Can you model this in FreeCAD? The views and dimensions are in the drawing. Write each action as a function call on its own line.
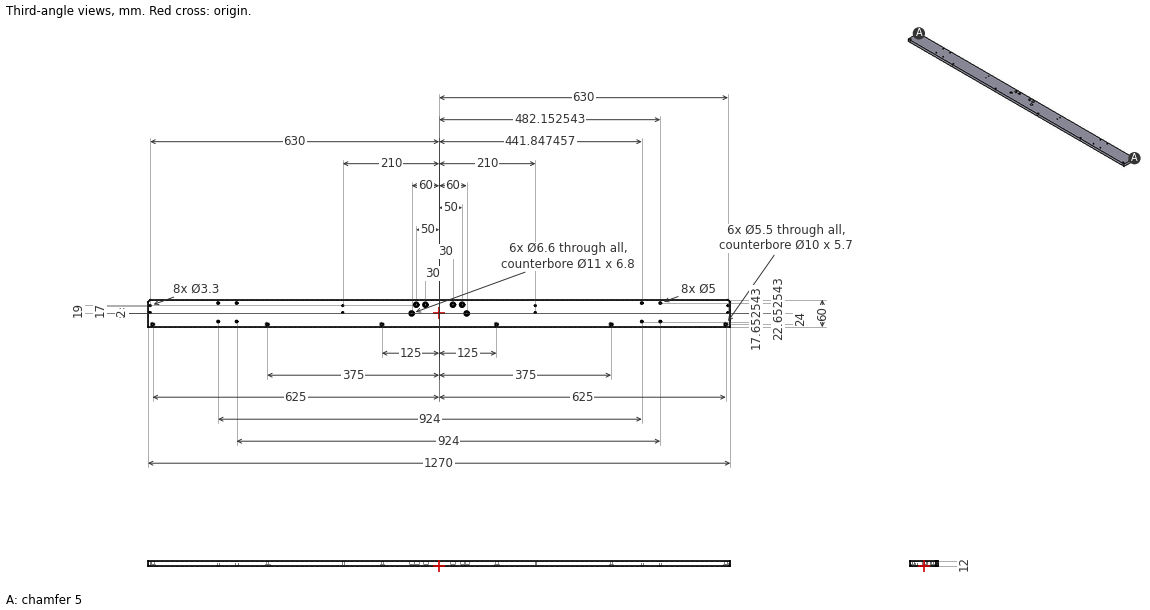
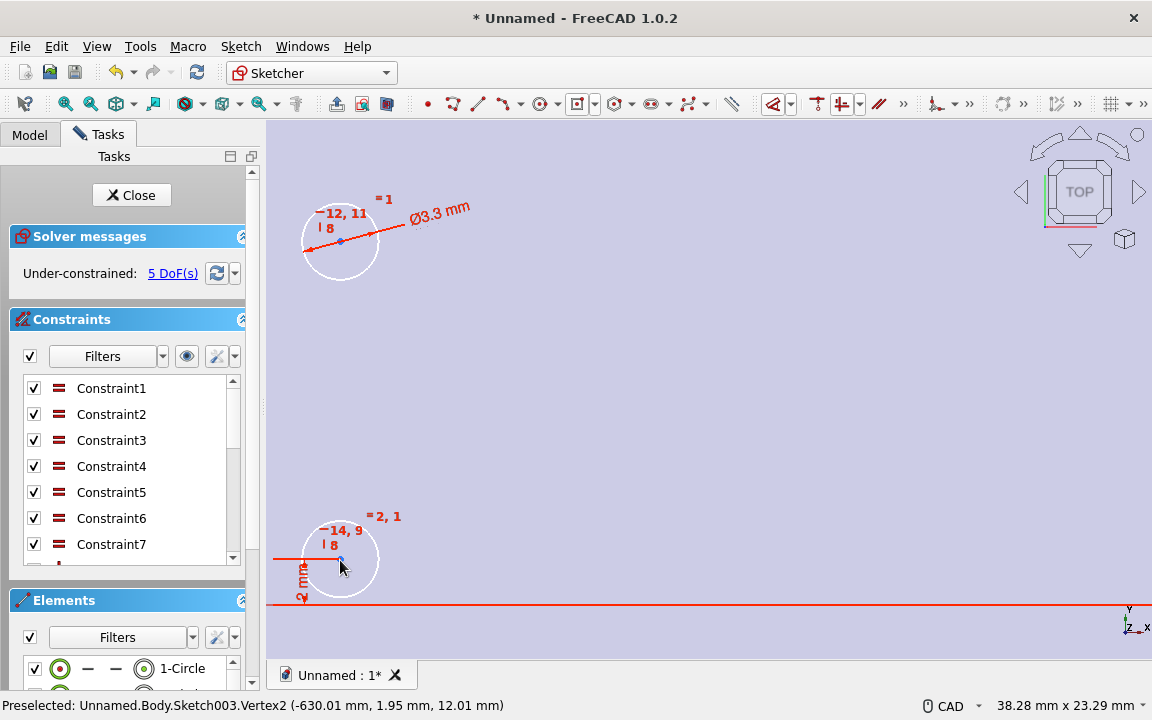
scroll(640, 390, down, 15)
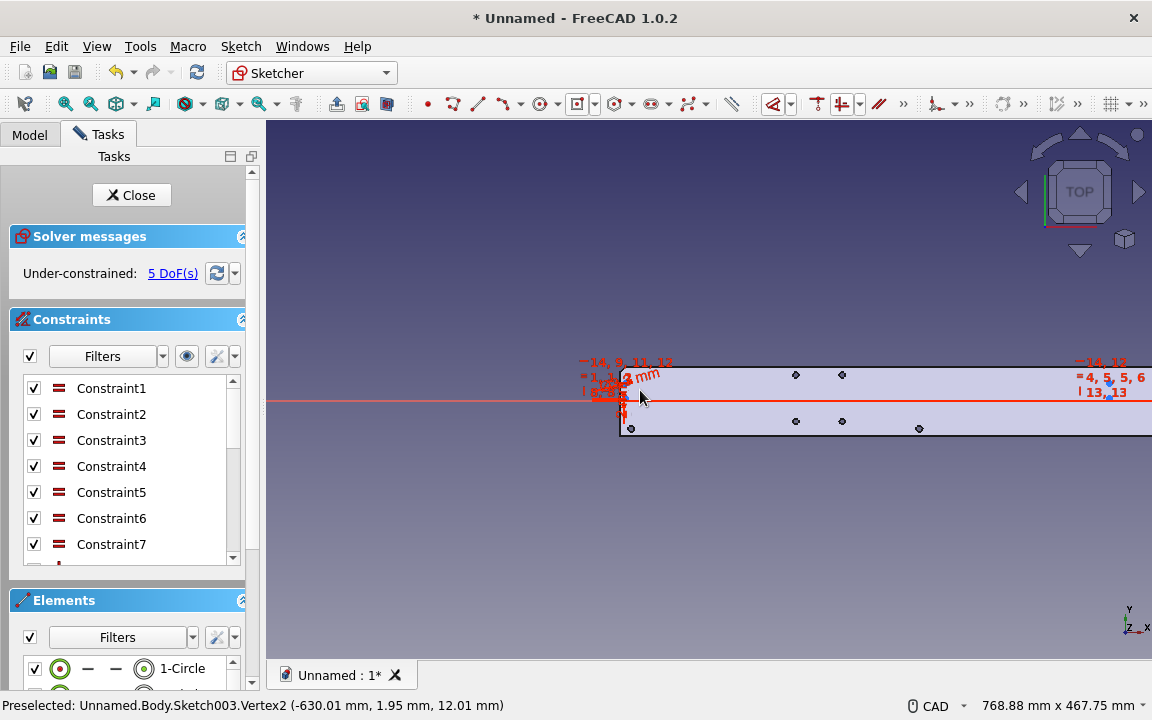
scroll(294, 389, down, 5)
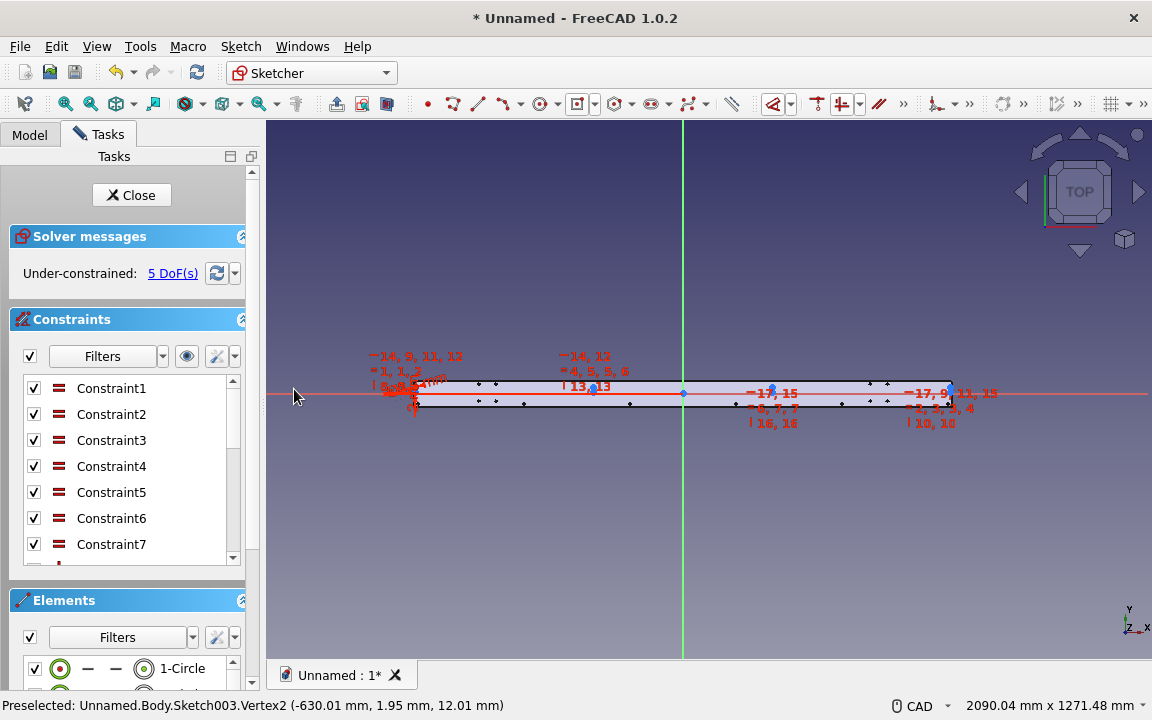
scroll(416, 387, up, 9)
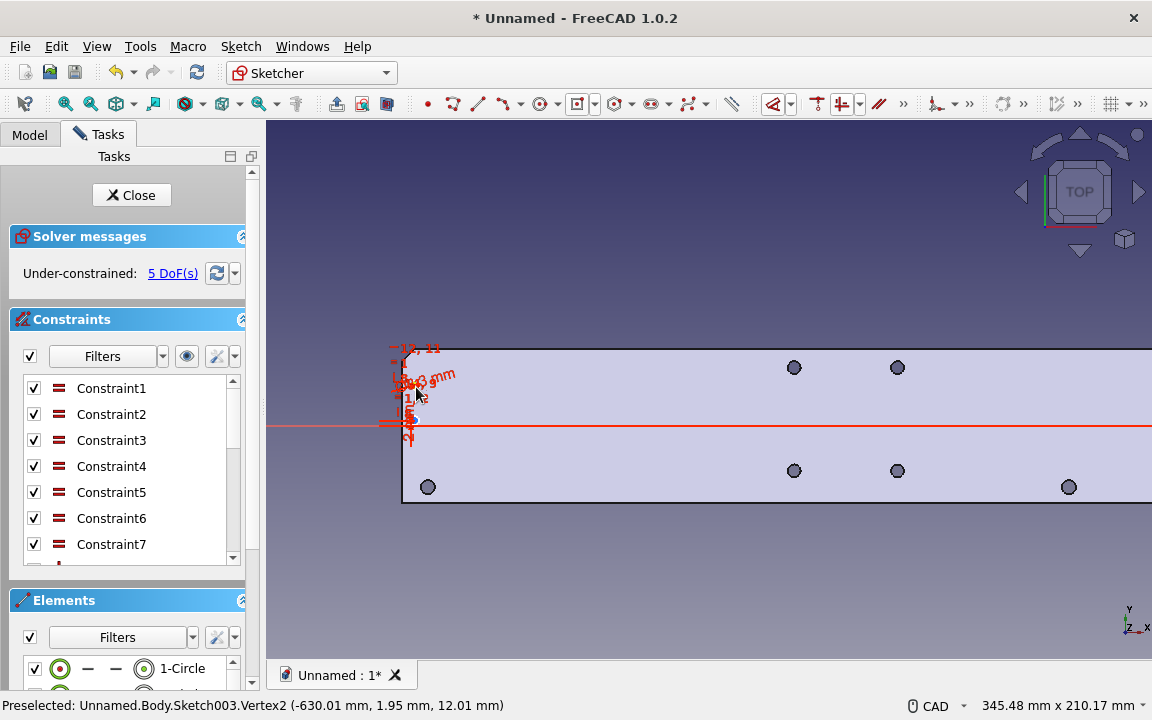
click(415, 385)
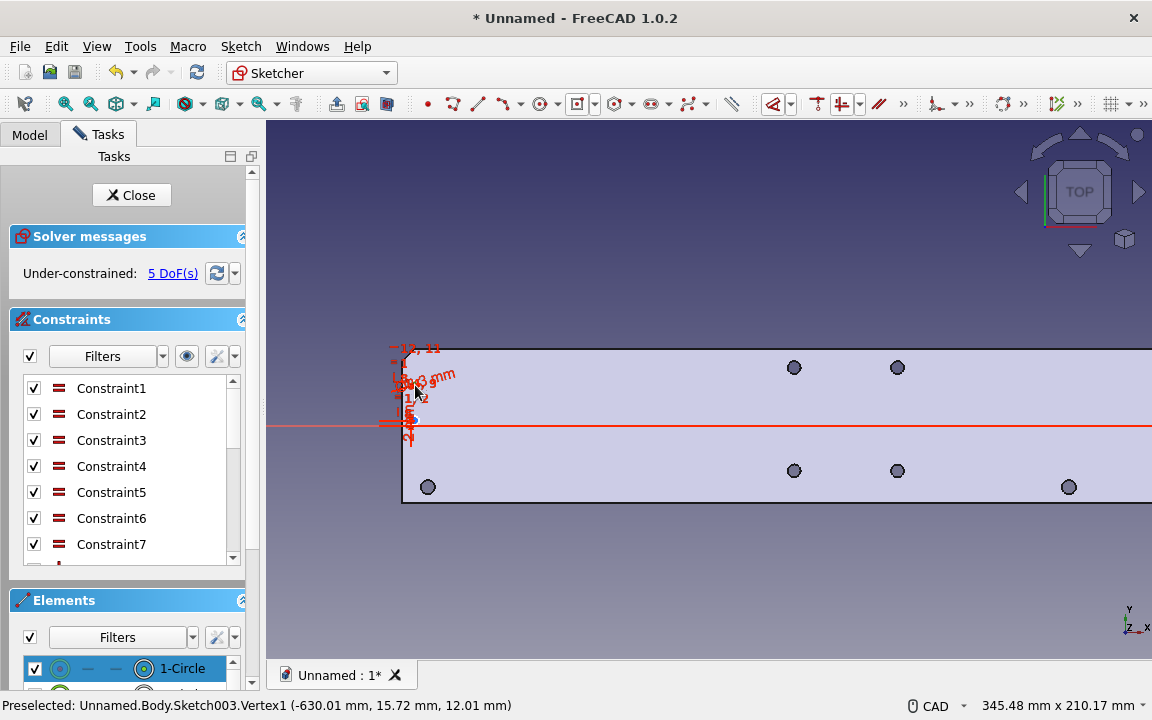
key(i)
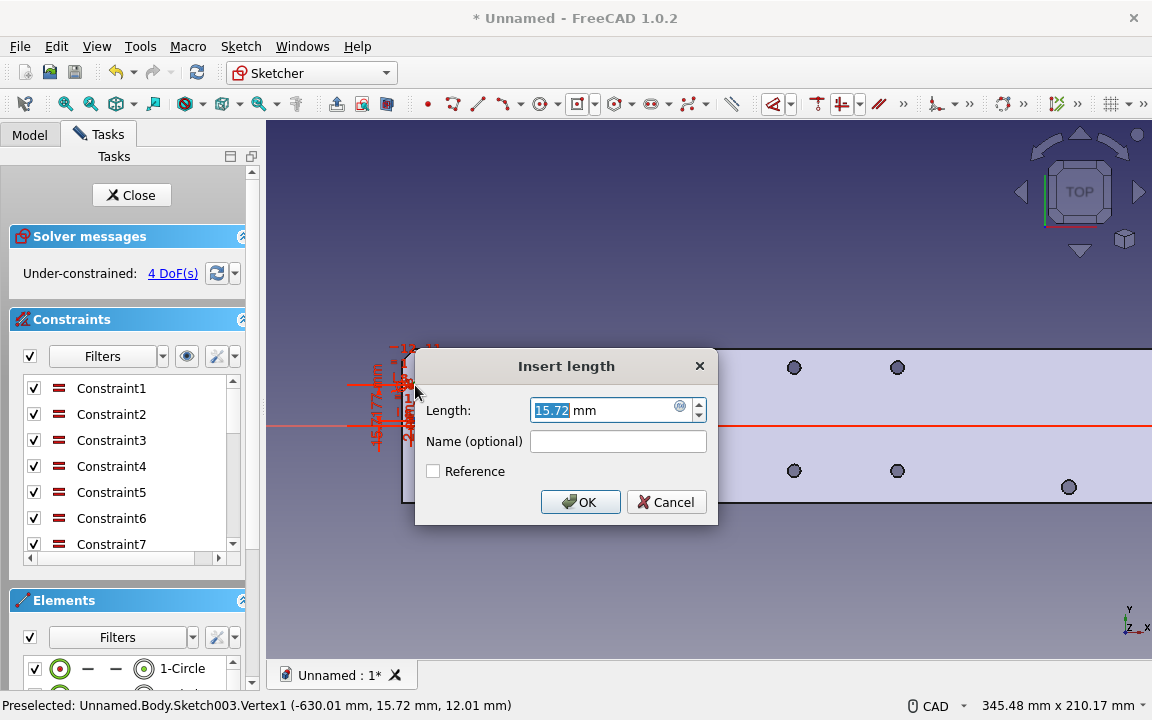
text(17)
key(Return)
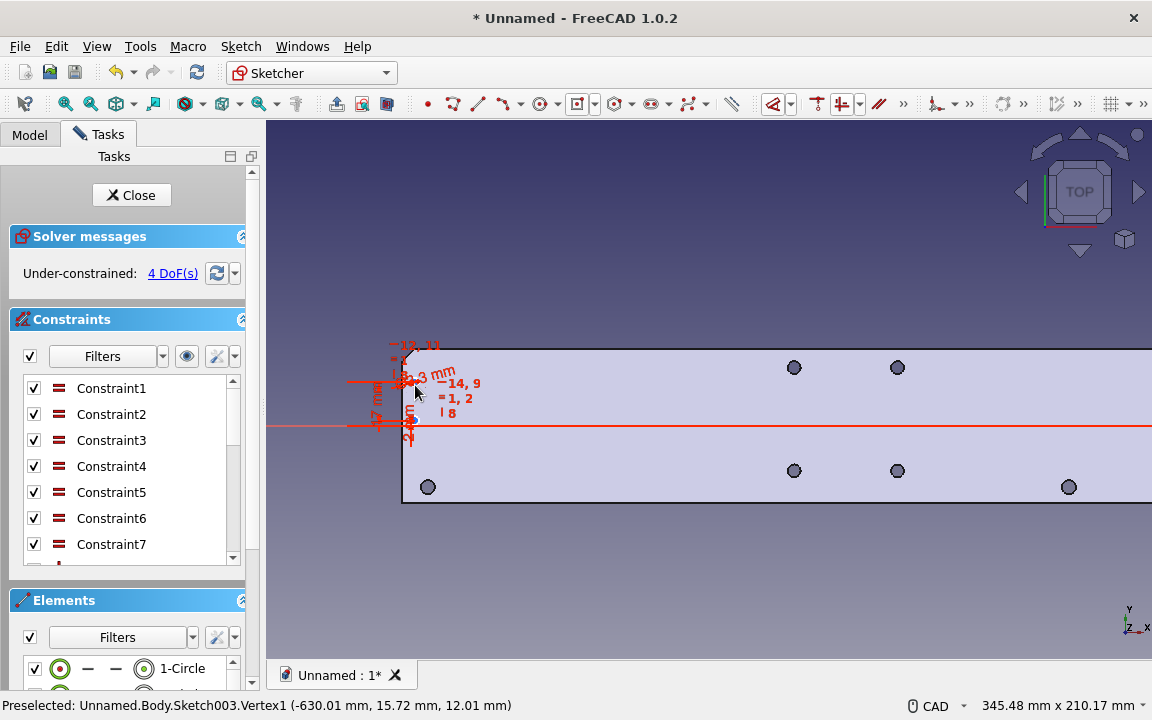
scroll(365, 387, down, 9)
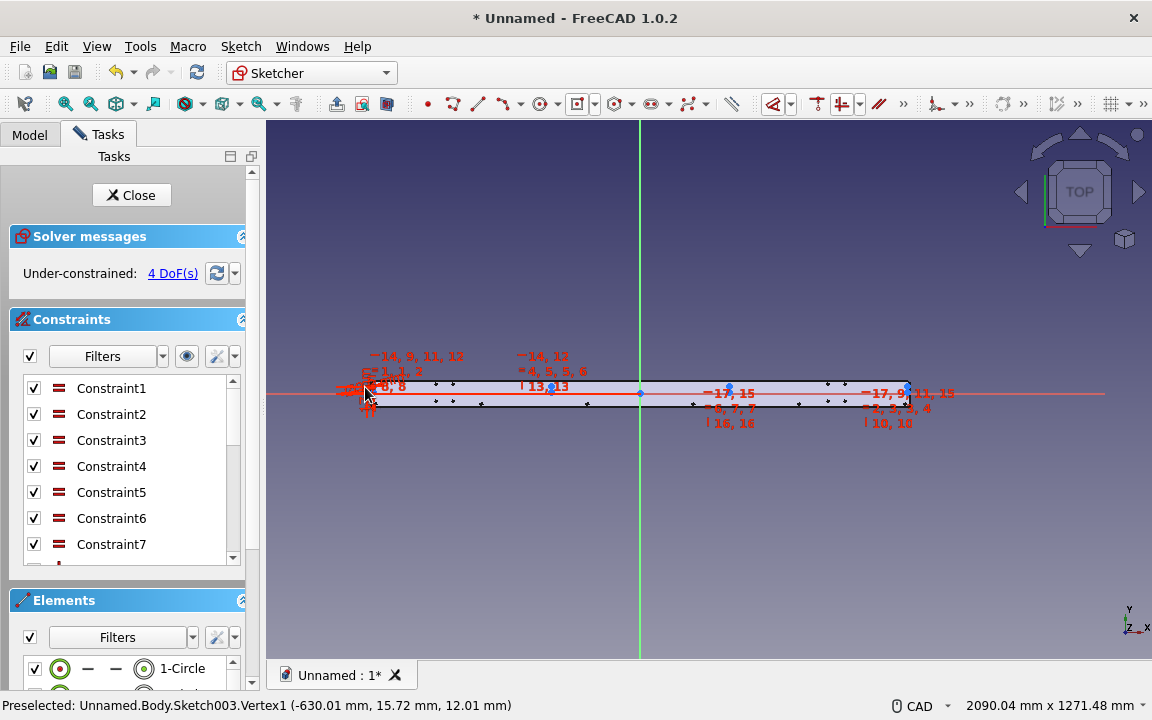
scroll(373, 387, up, 4)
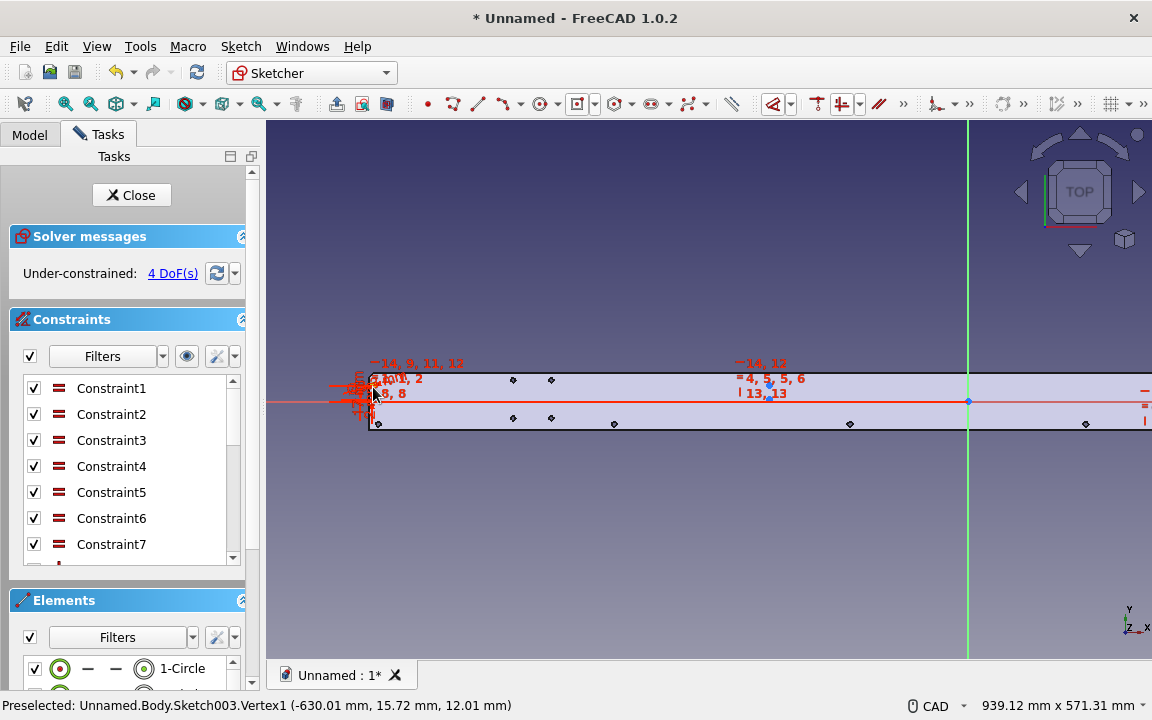
click(374, 385)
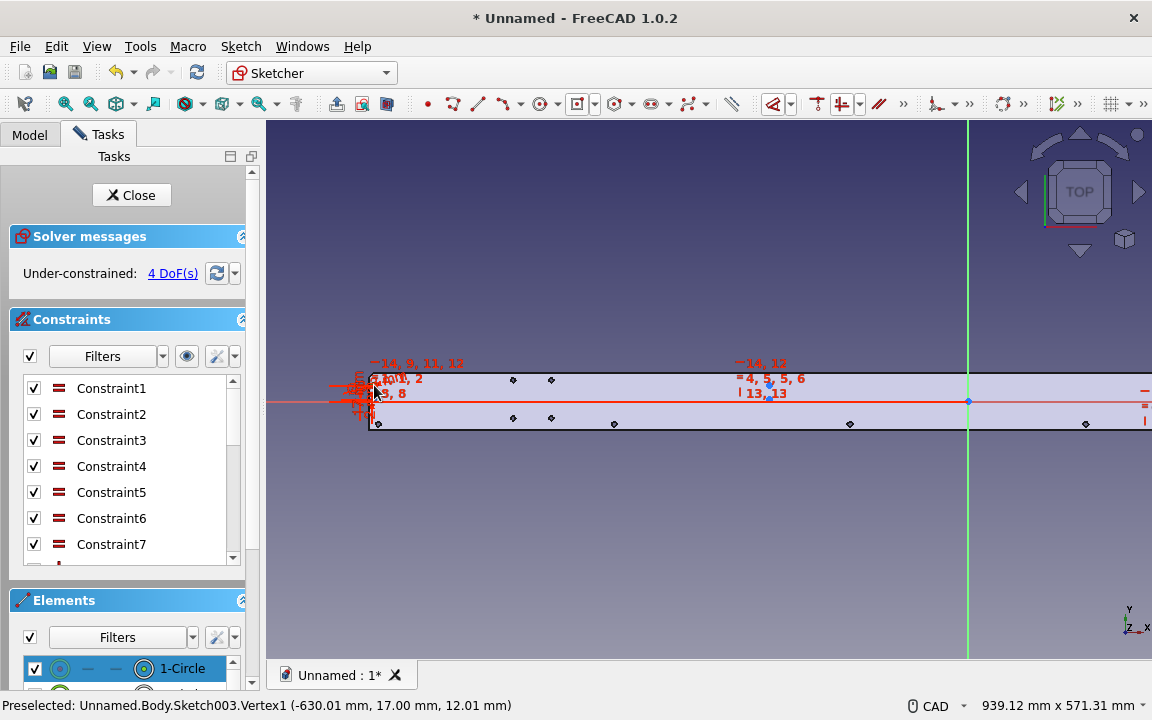
key(l)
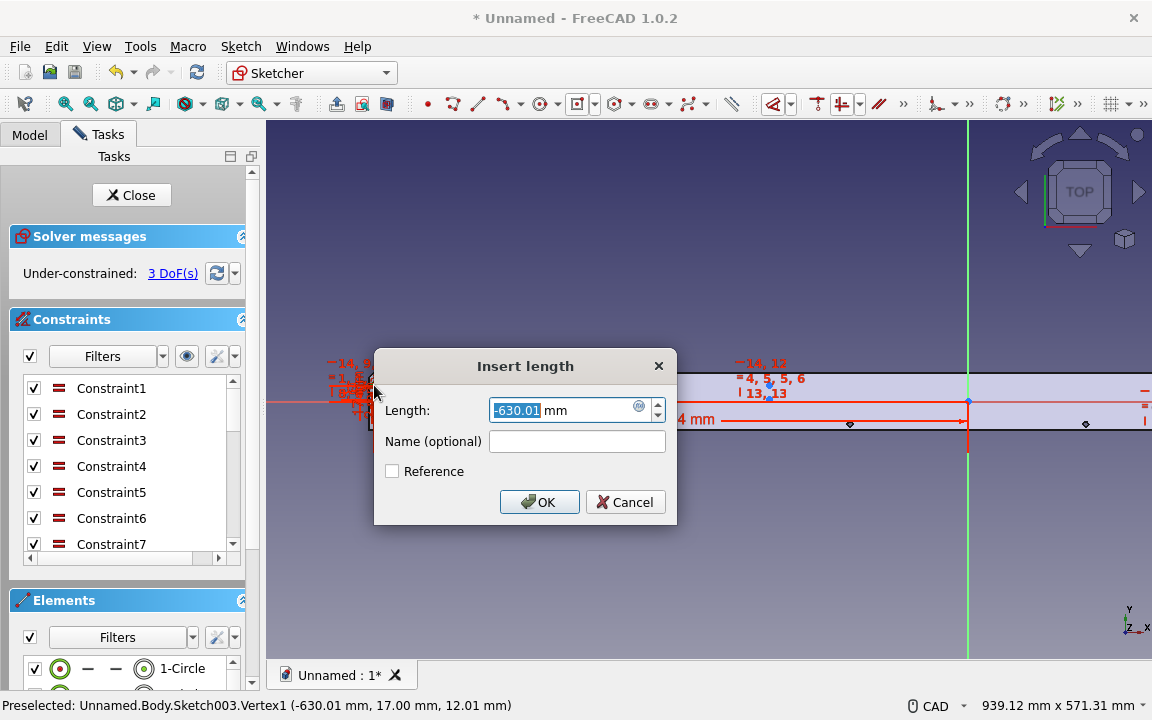
text(-630)
key(Return)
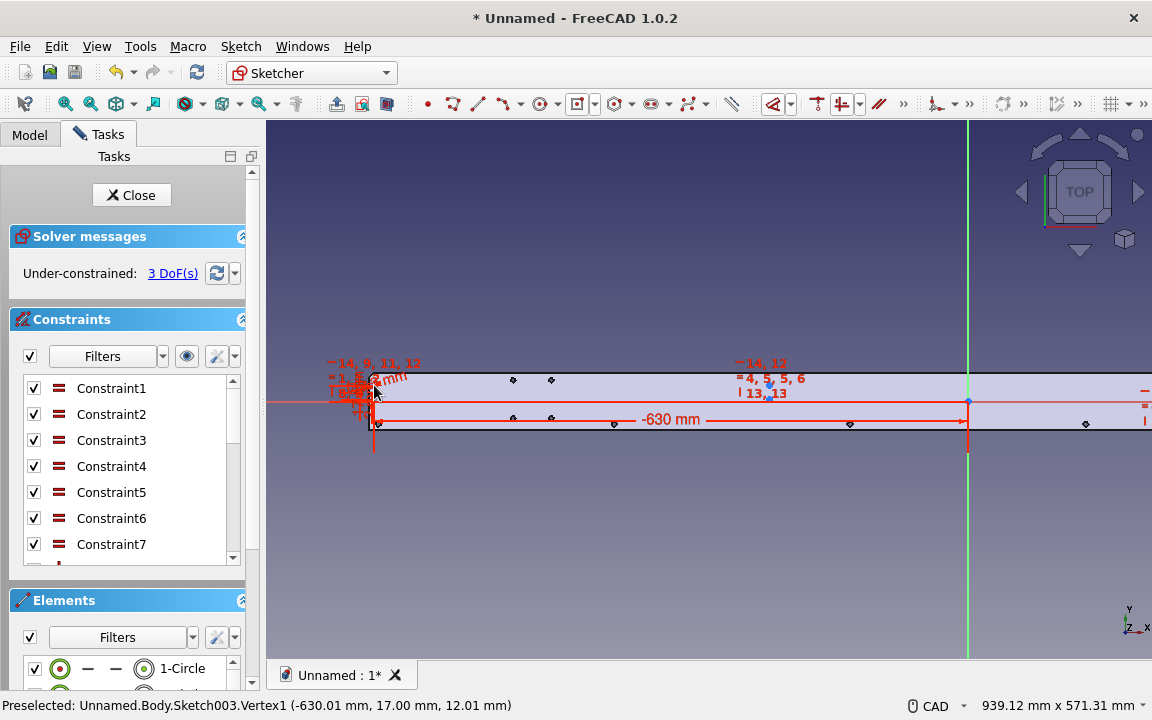
scroll(373, 387, down, 4)